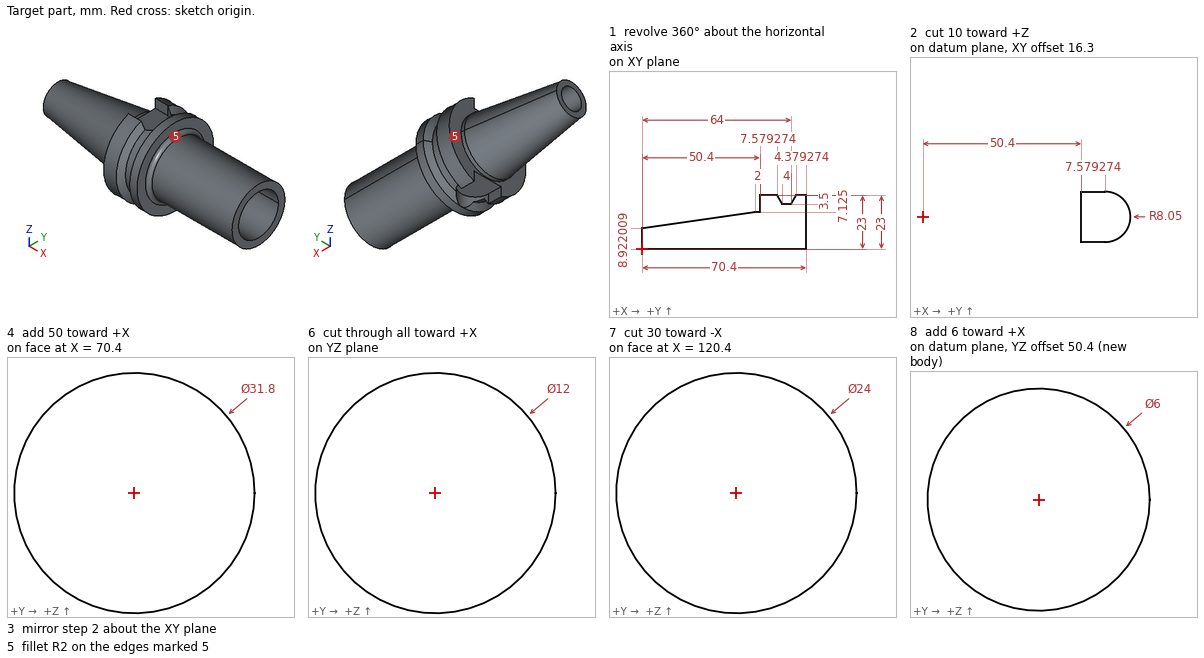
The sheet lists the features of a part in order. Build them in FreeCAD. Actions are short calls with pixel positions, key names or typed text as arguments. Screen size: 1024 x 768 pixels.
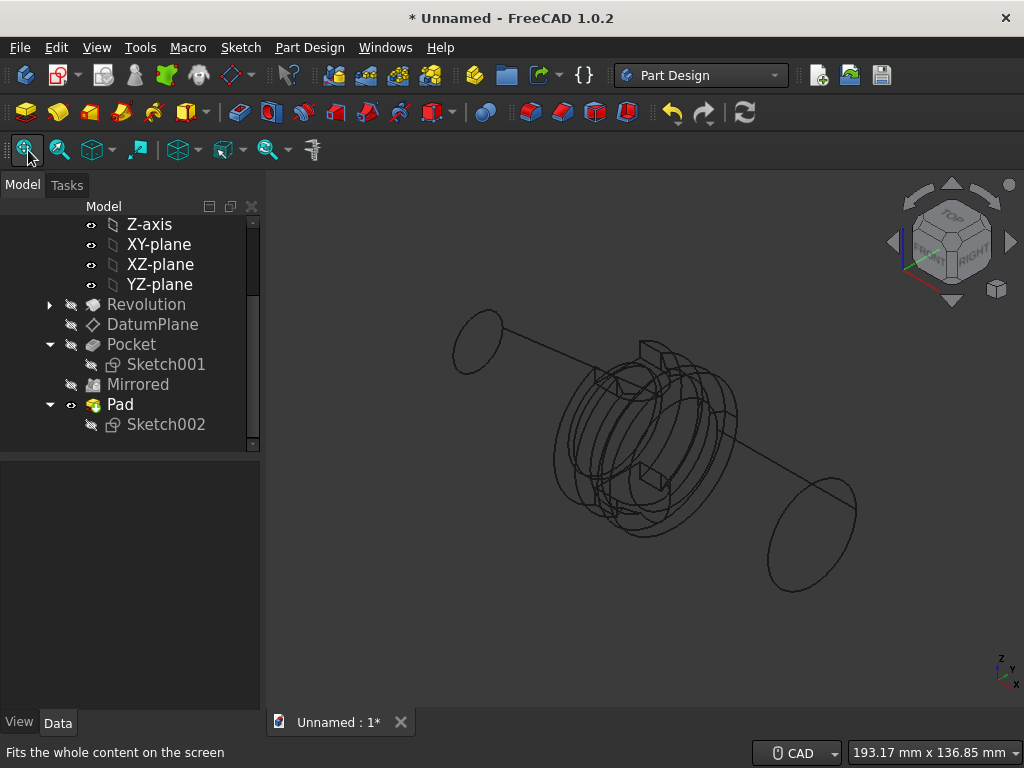
click(629, 479)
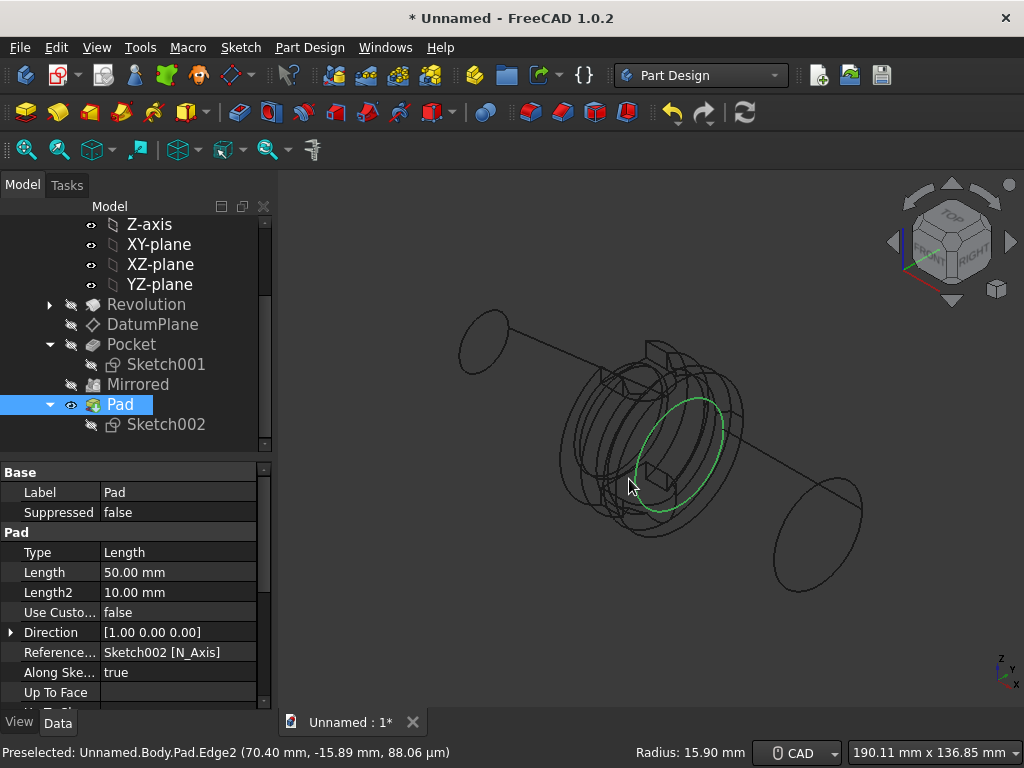
key(v)
key(1)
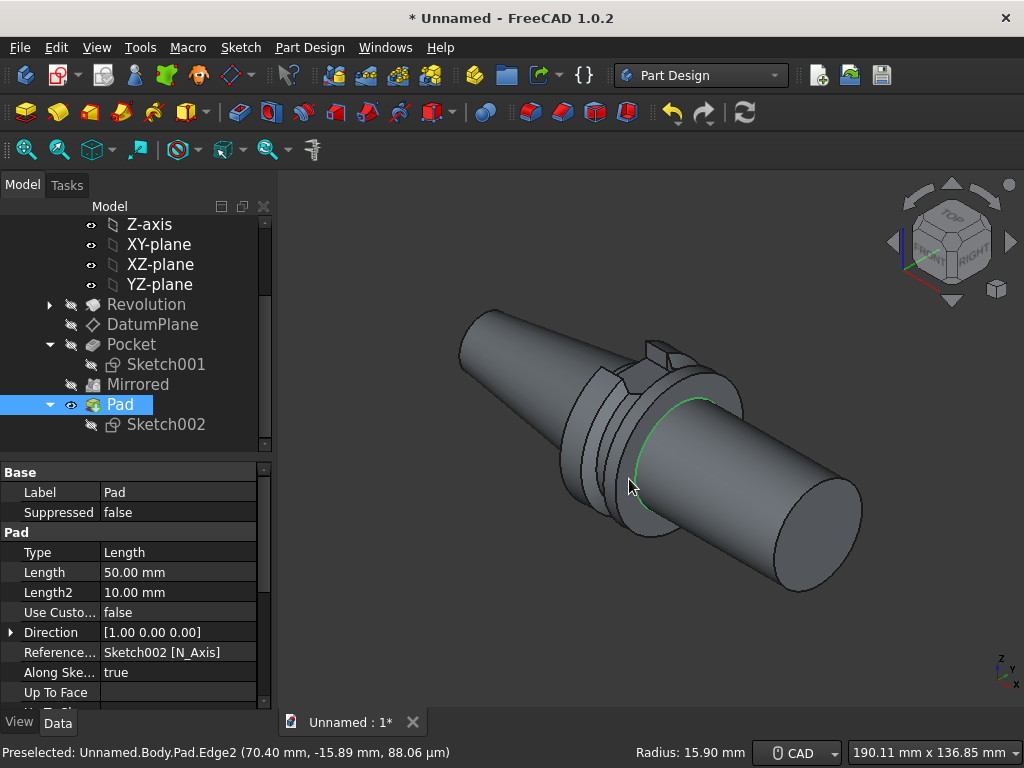
click(532, 112)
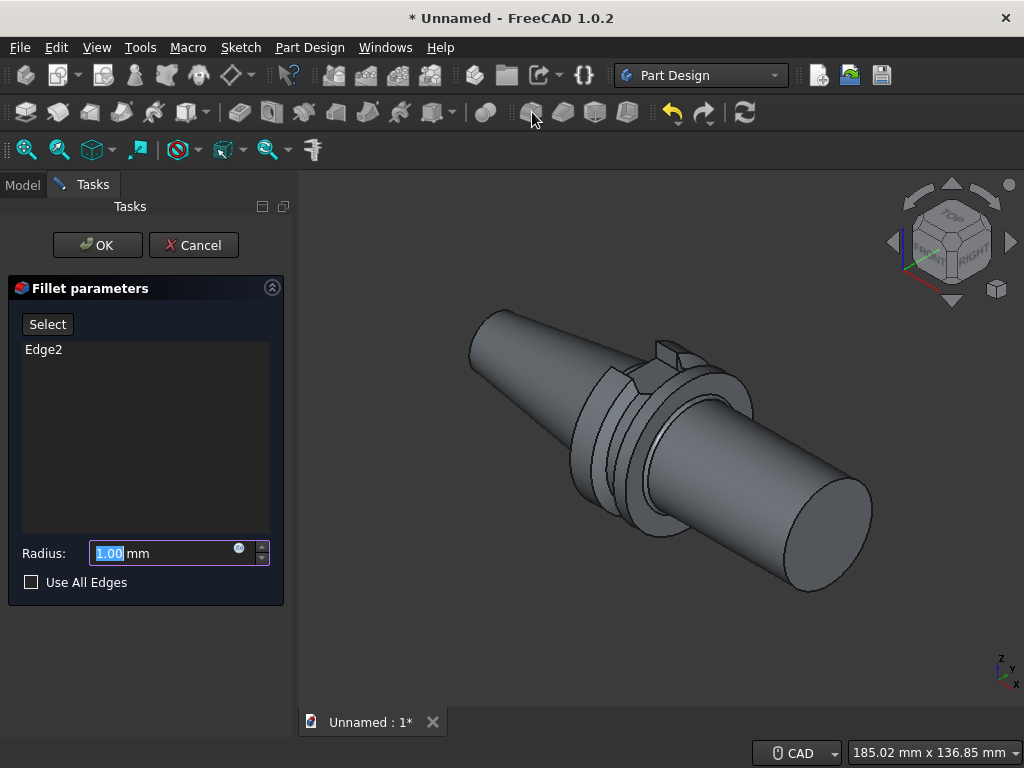
text(2)
key(Tab)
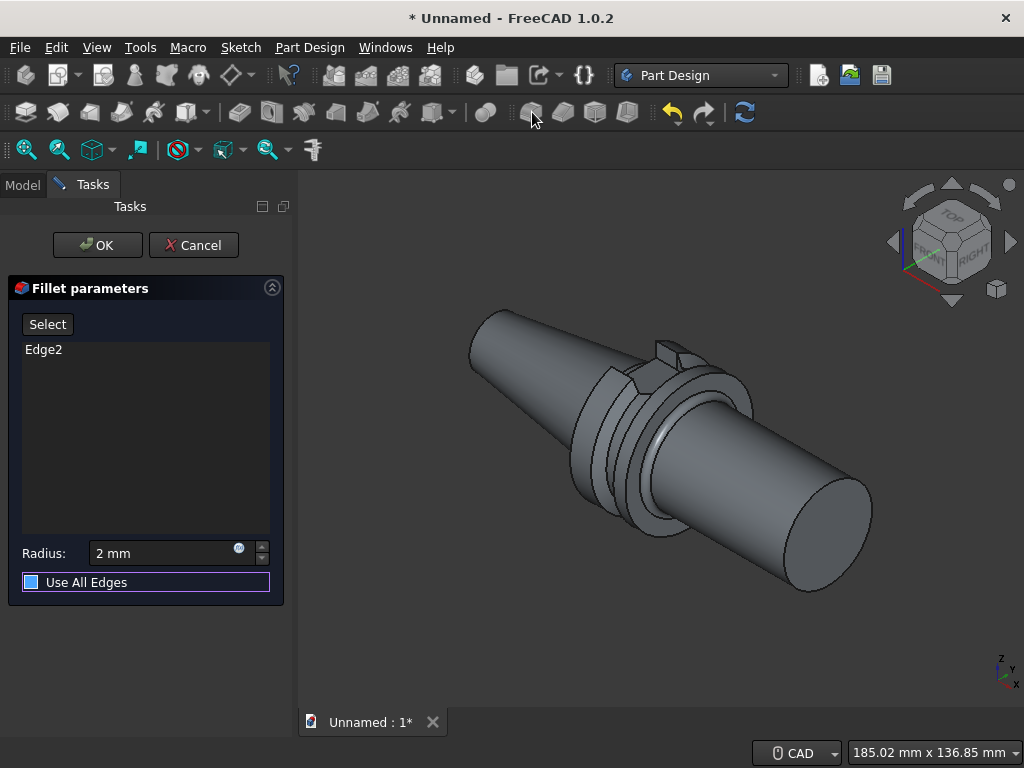
click(98, 245)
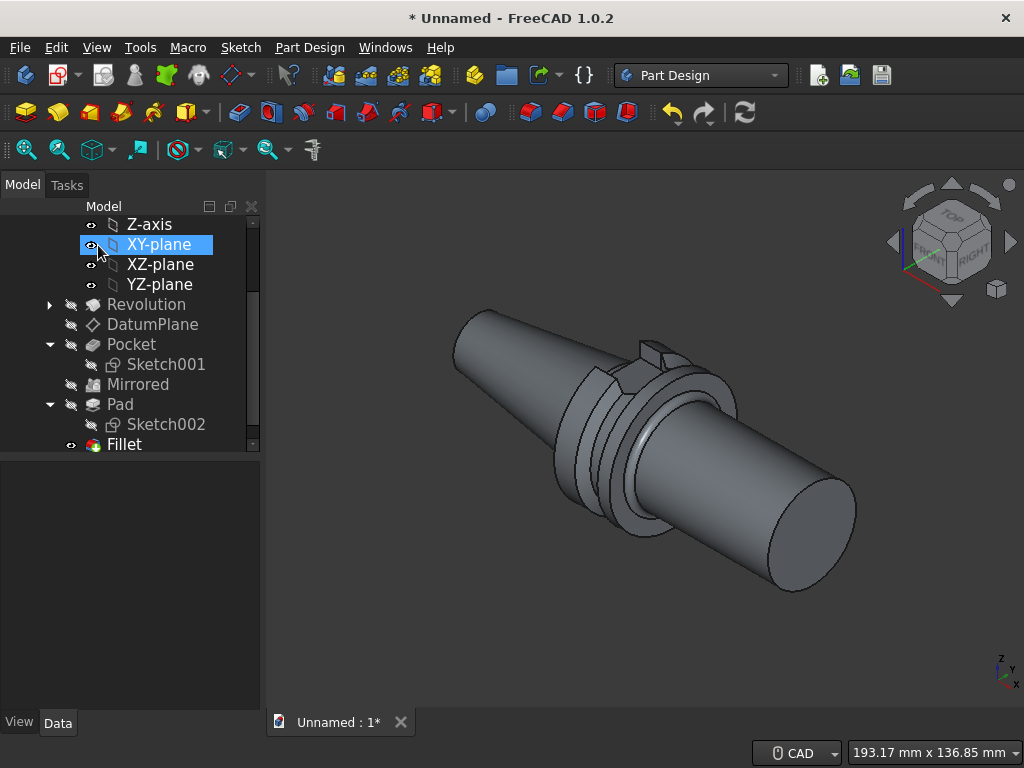
click(58, 76)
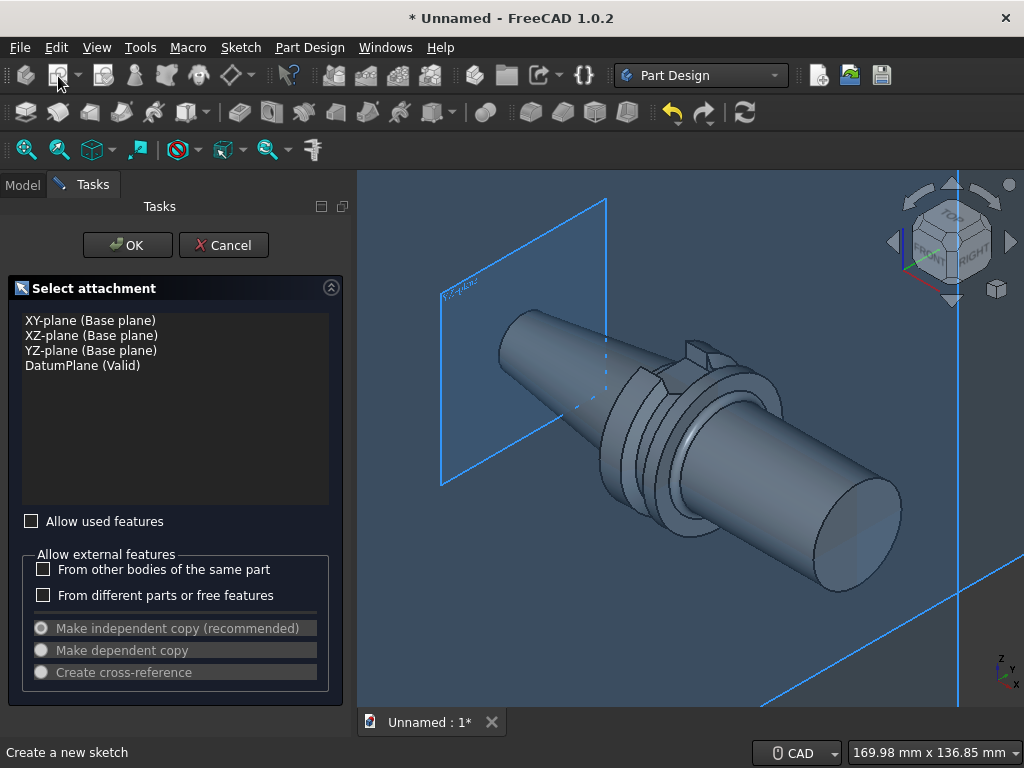
click(82, 350)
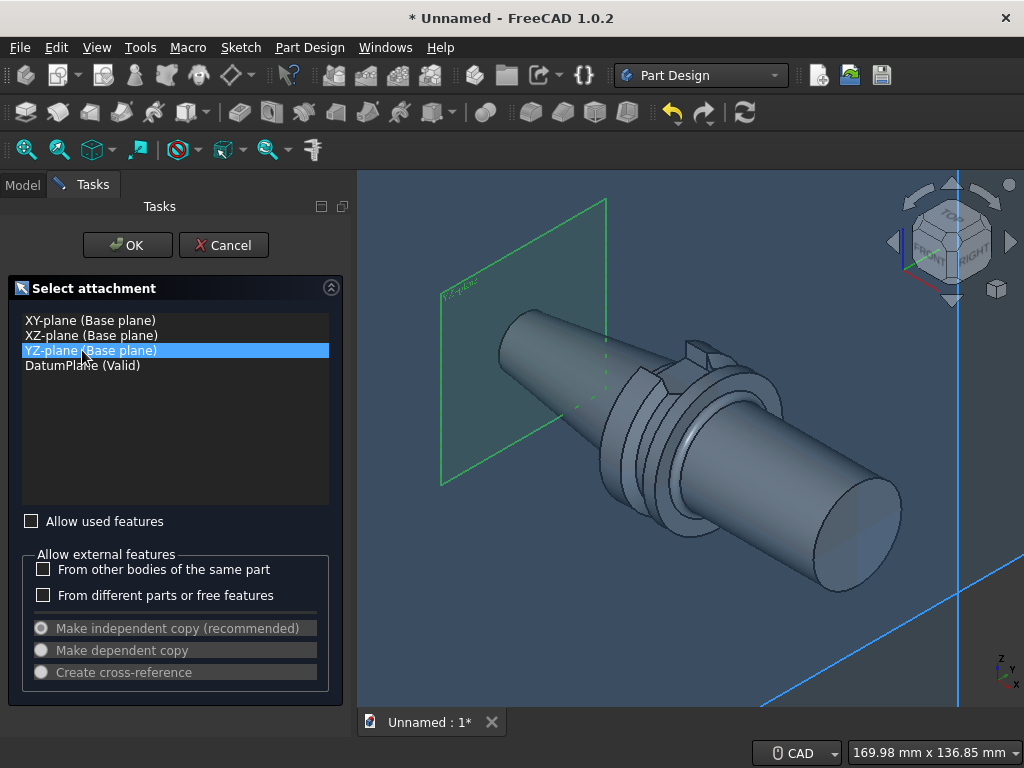
click(128, 245)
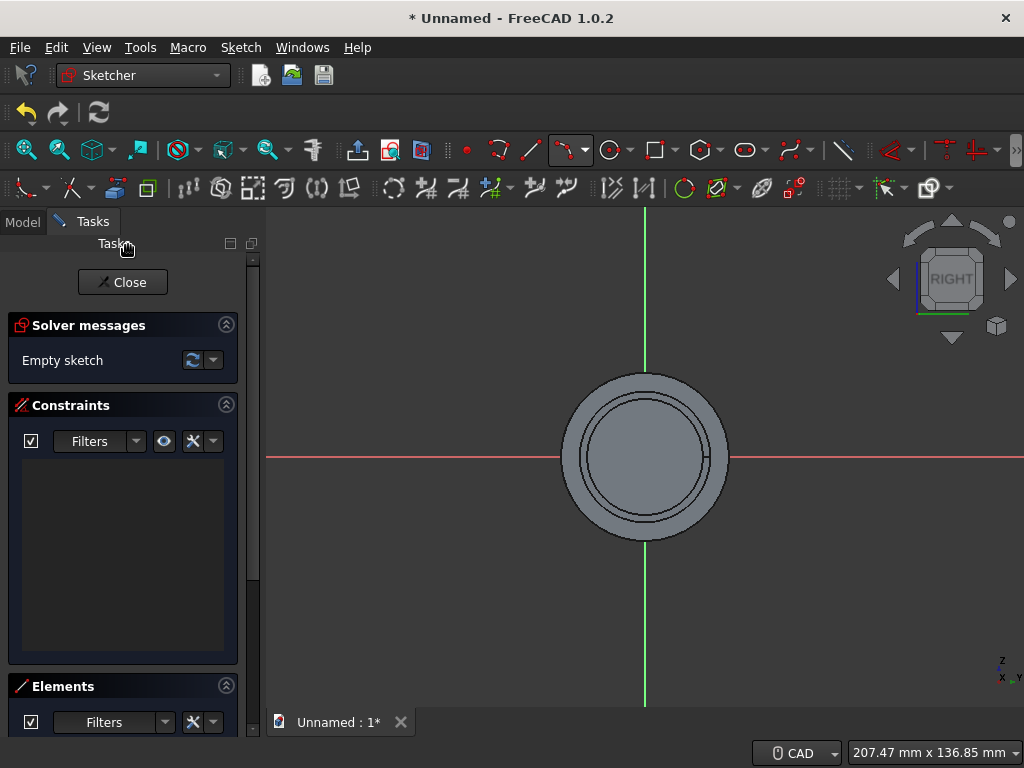
key(q)
key(s)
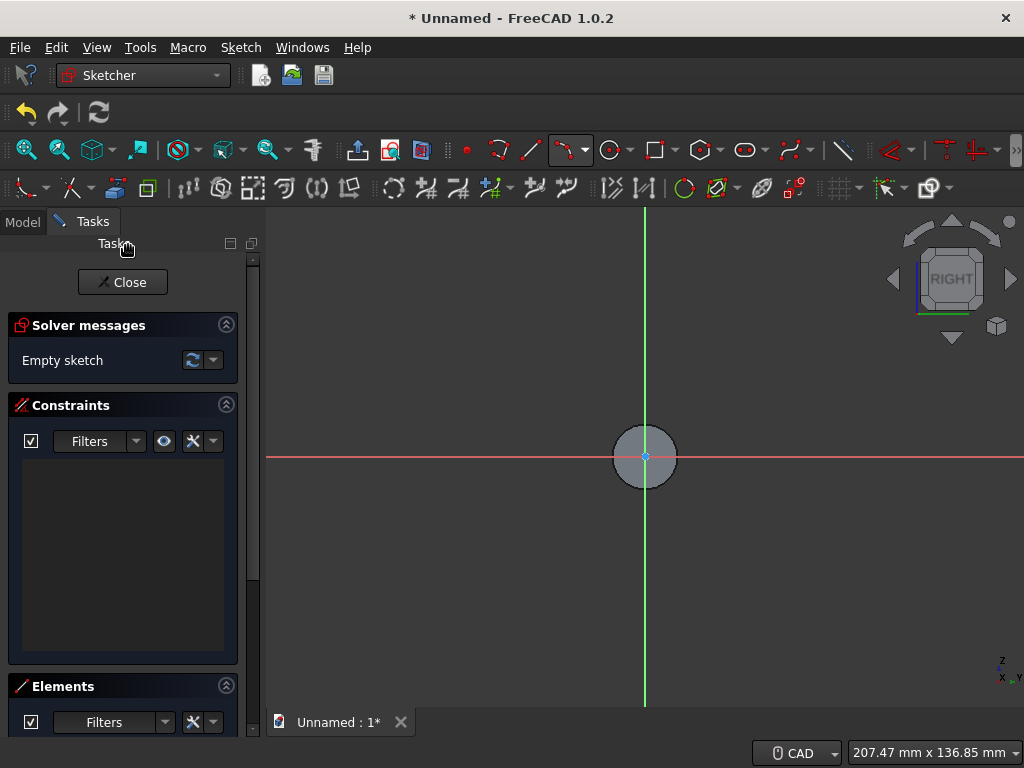
scroll(656, 457, up, 10)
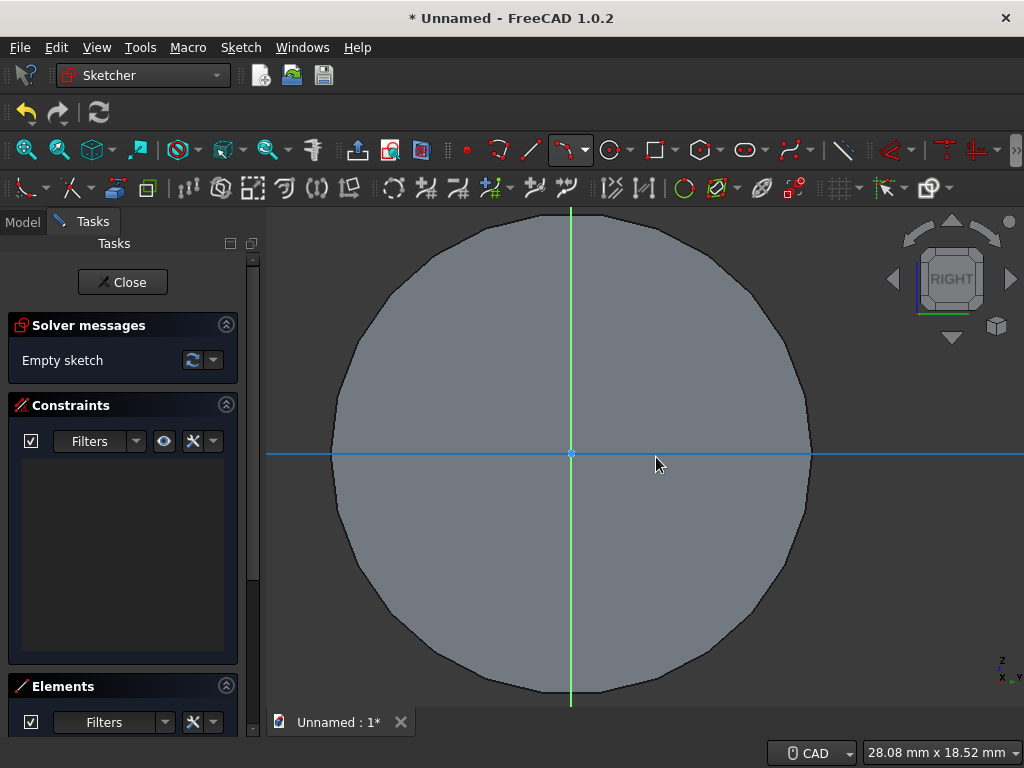
click(610, 150)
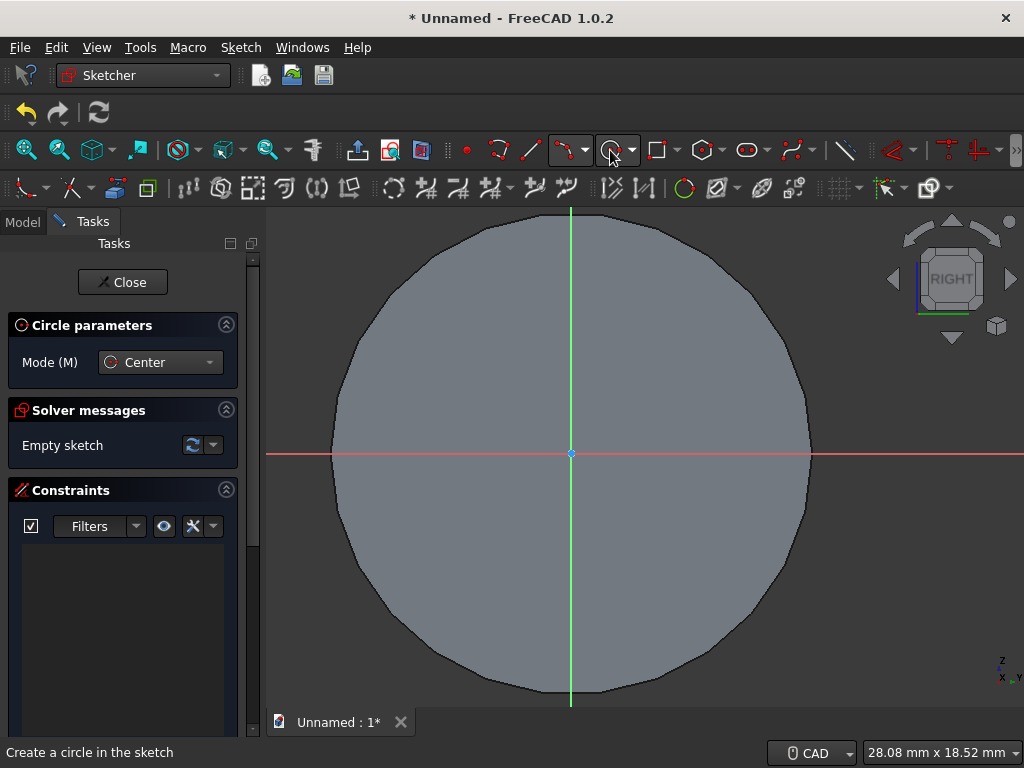
click(571, 454)
move(686, 339)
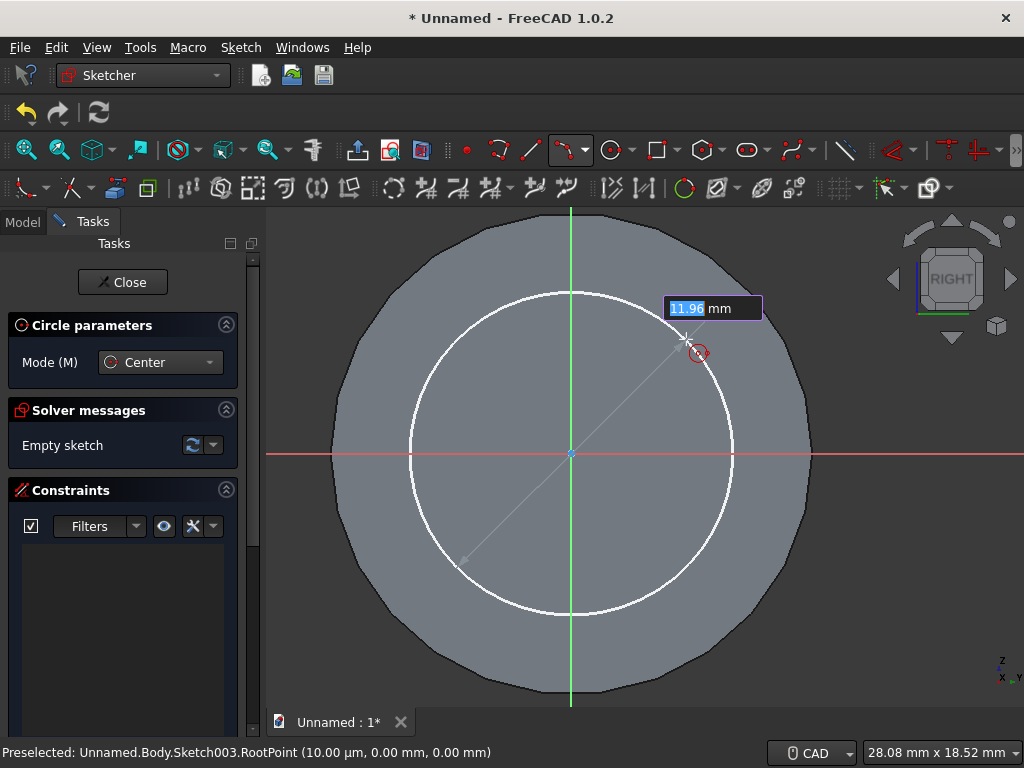
text(12)
key(Return)
key(Escape)